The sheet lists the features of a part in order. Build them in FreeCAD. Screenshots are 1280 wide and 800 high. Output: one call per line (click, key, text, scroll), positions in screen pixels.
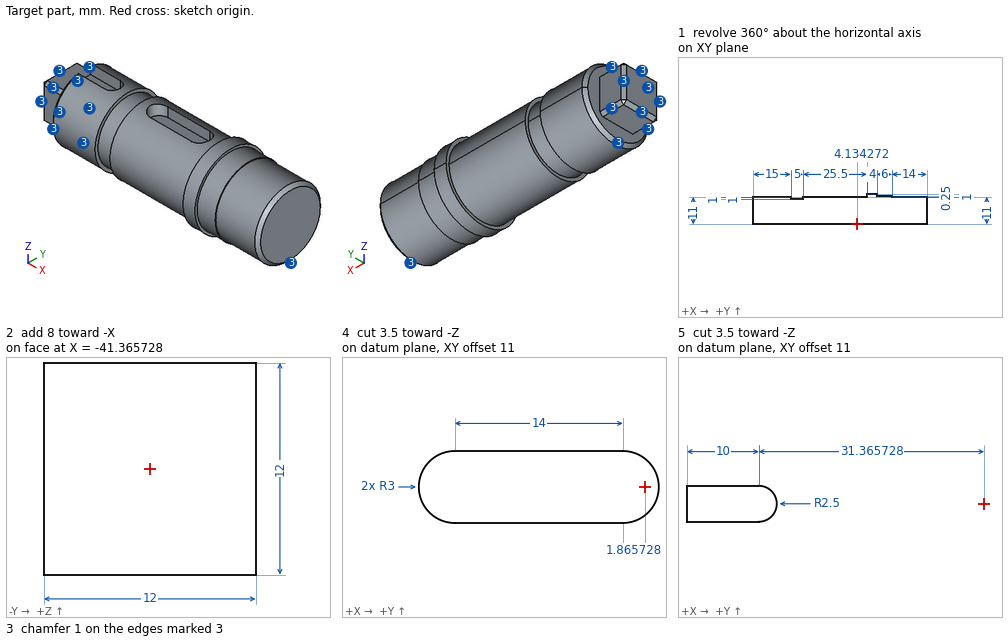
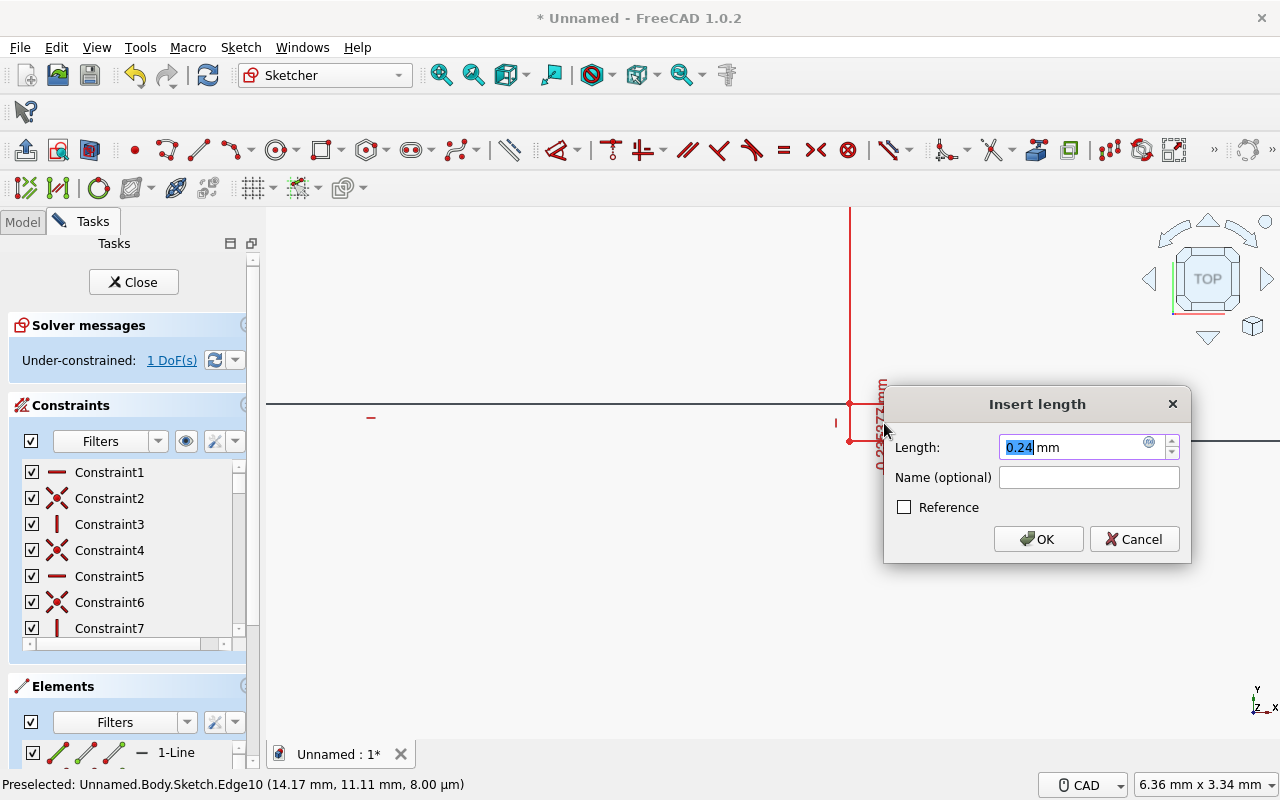
text(0.25)
key(Return)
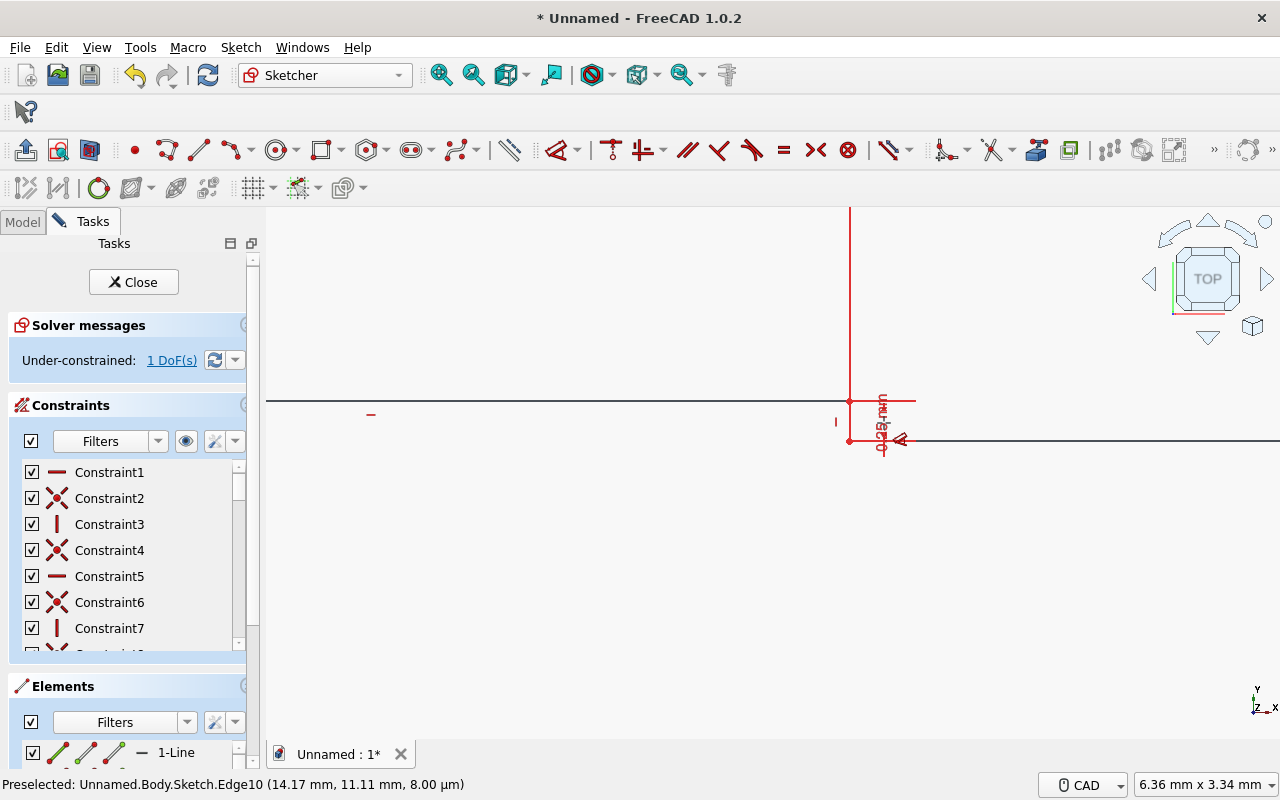
scroll(871, 433, down, 15)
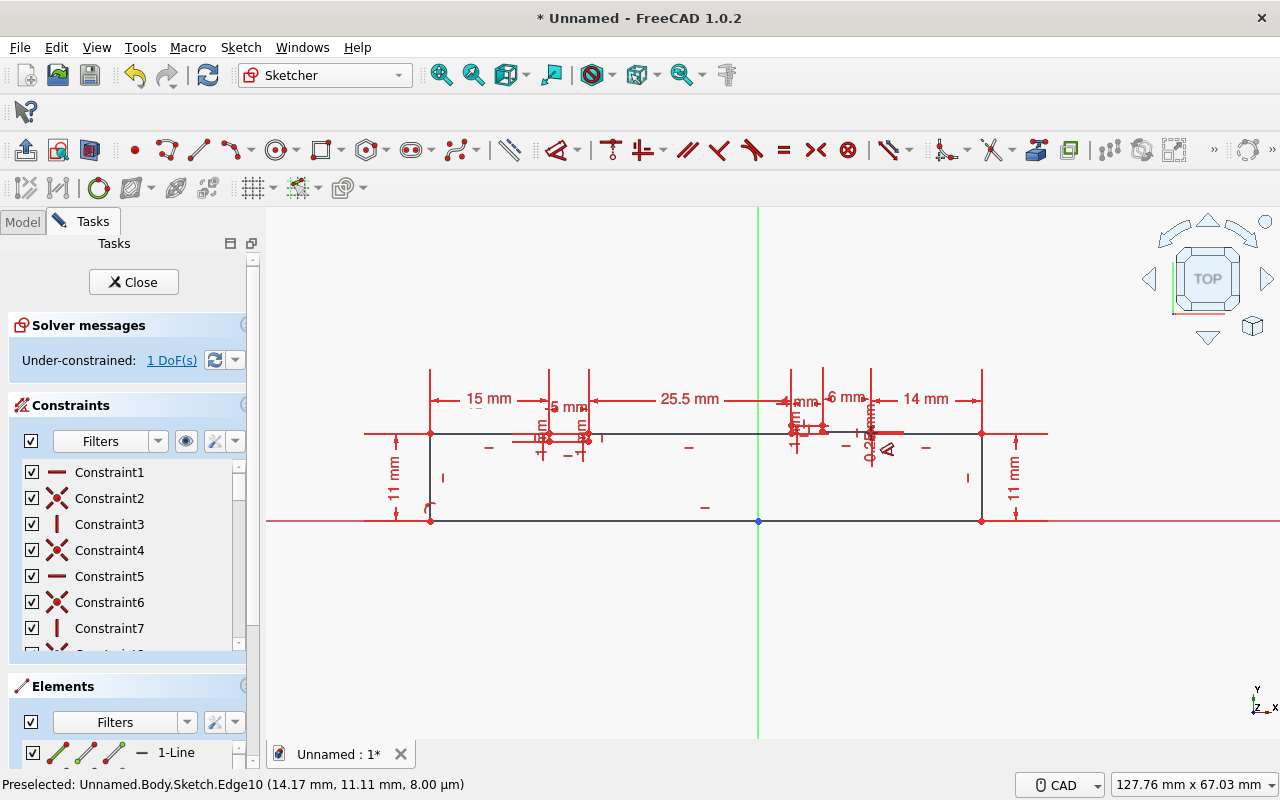
scroll(791, 434, up, 3)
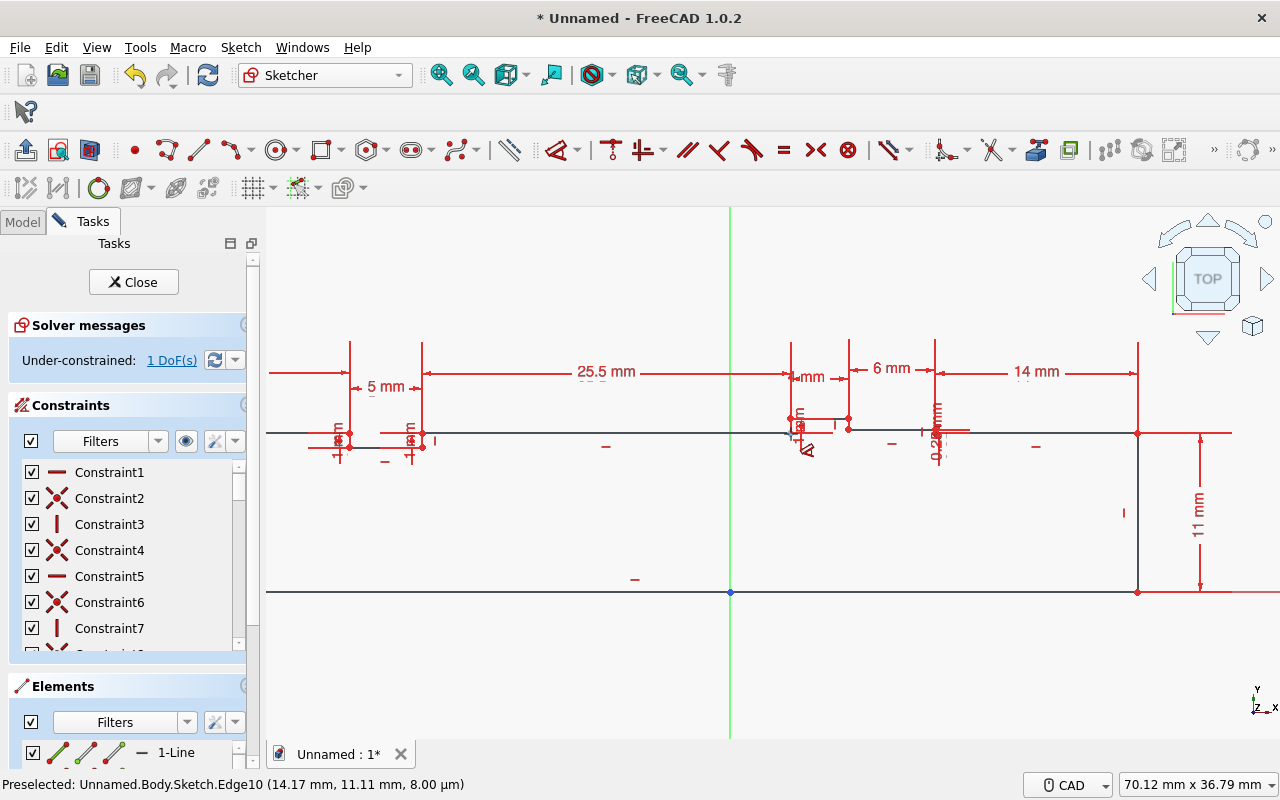
click(791, 433)
click(761, 626)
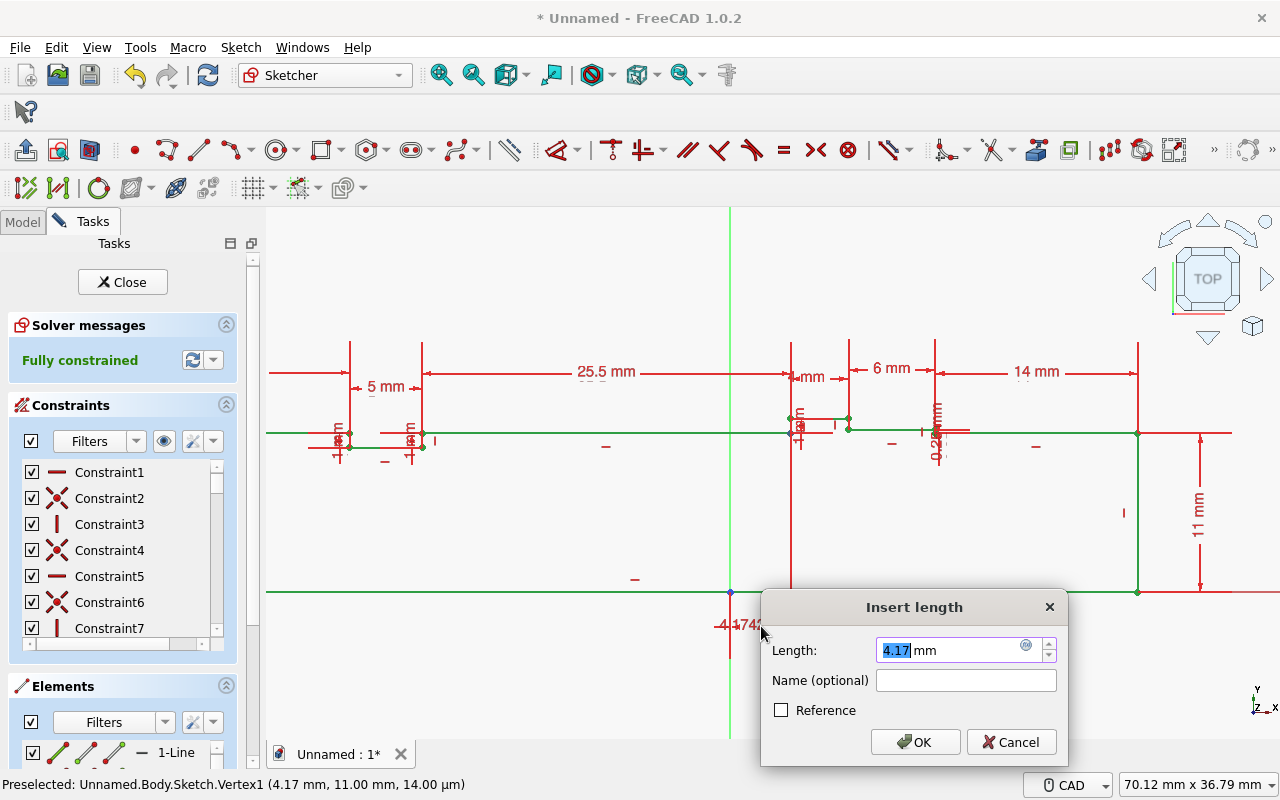
text(4.134272)
key(Return)
key(Escape)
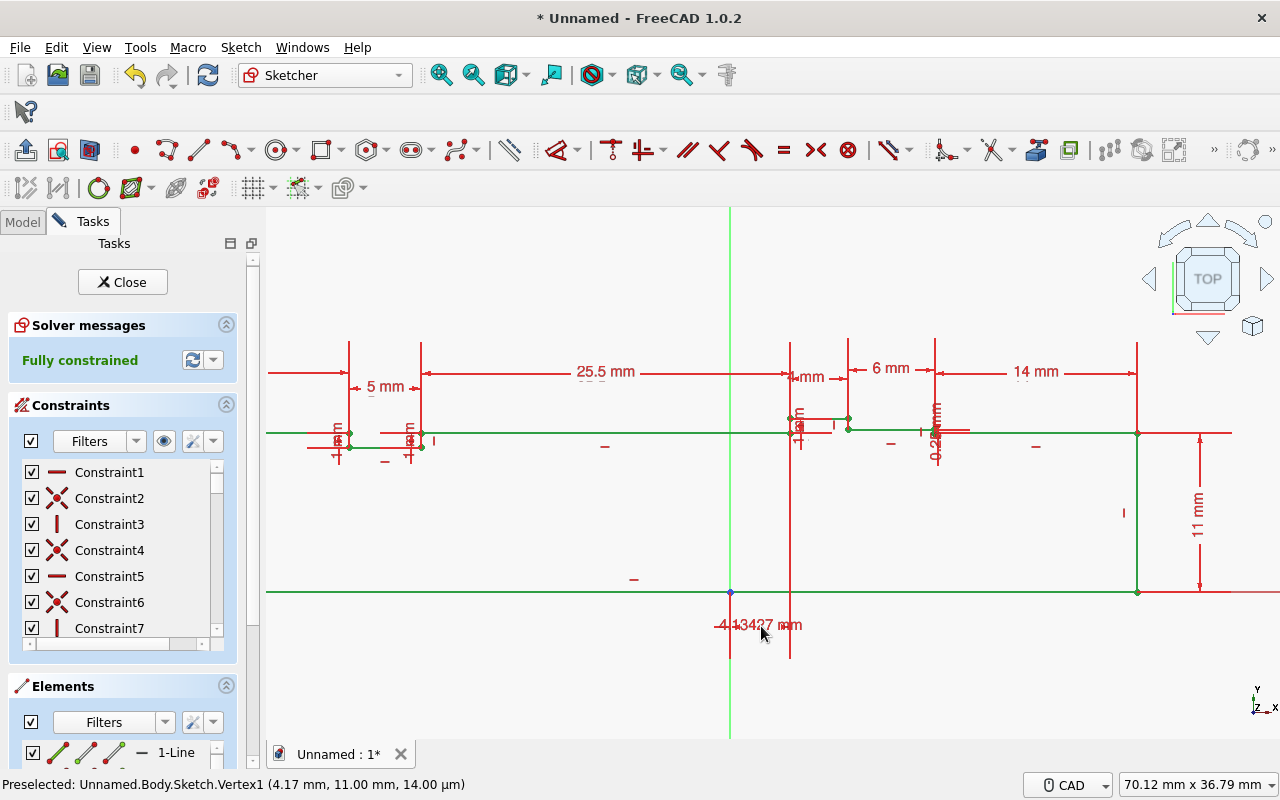
click(123, 282)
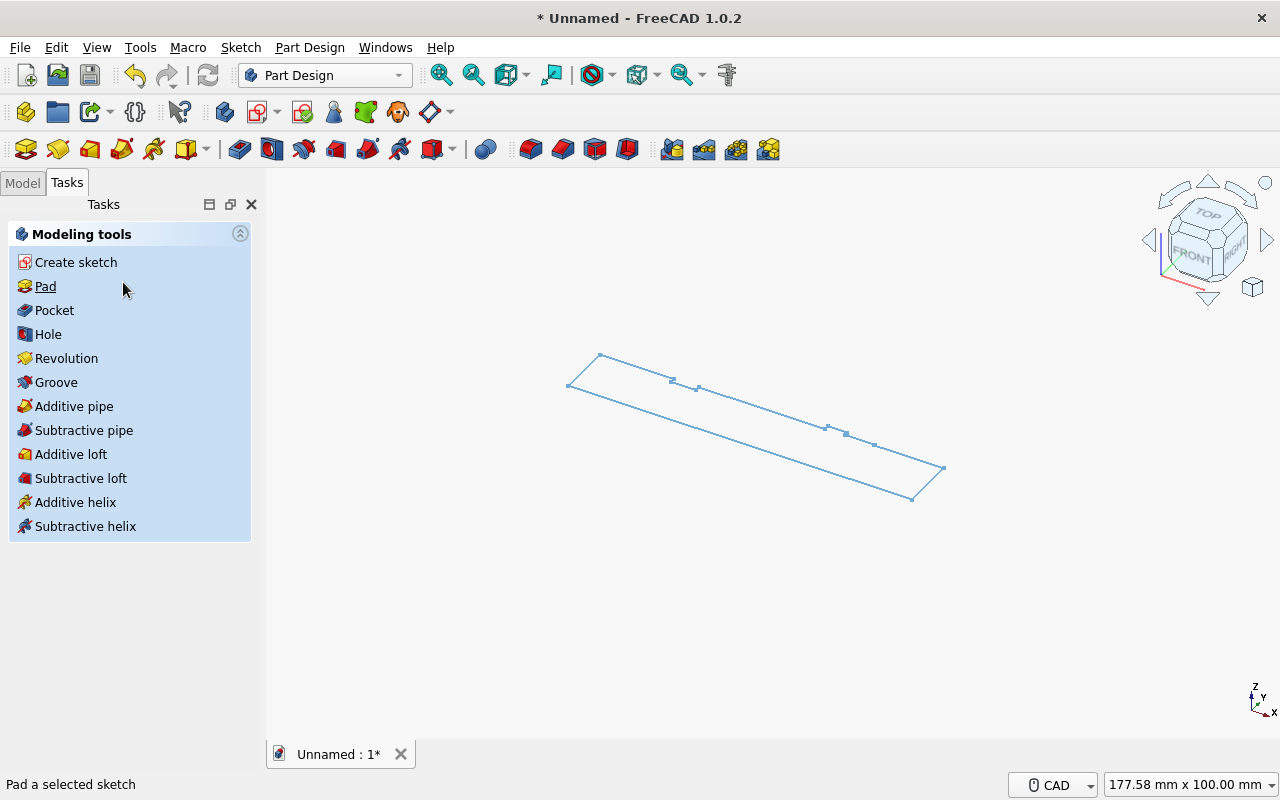
click(58, 150)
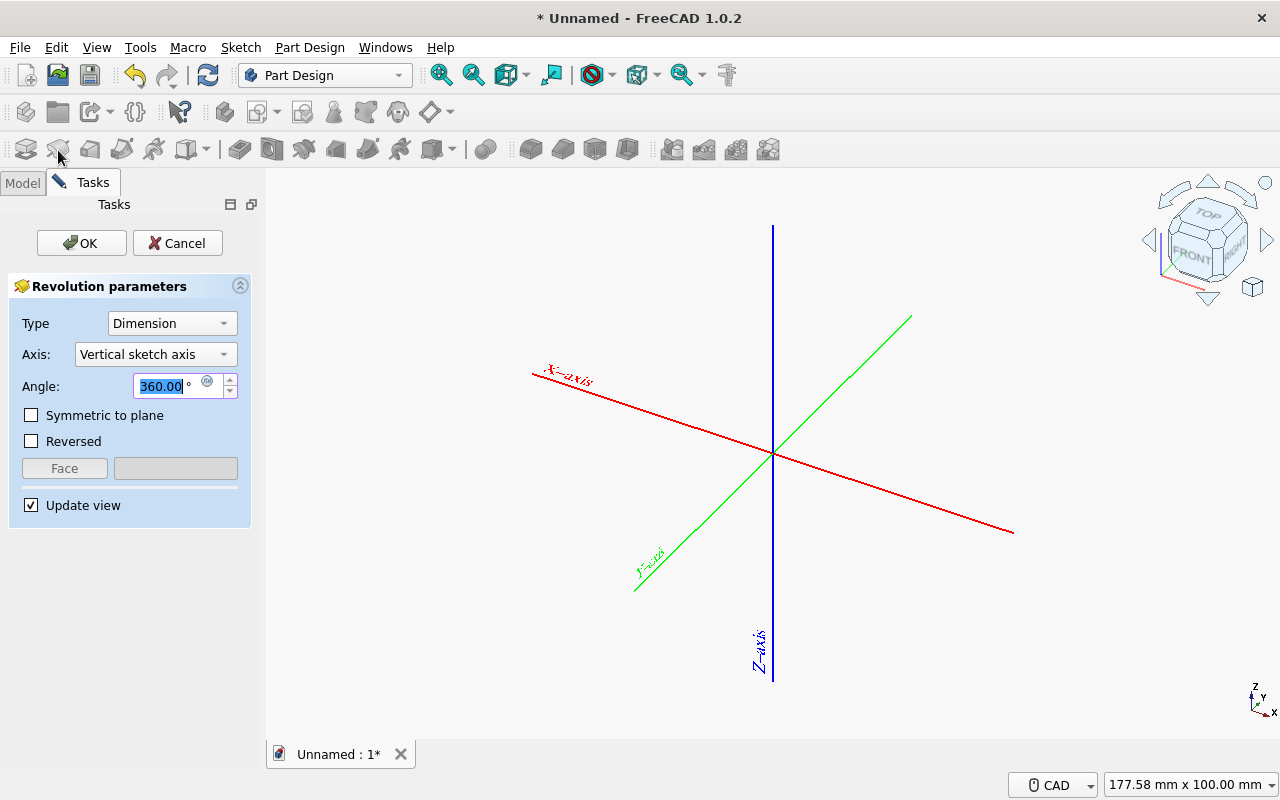
click(156, 354)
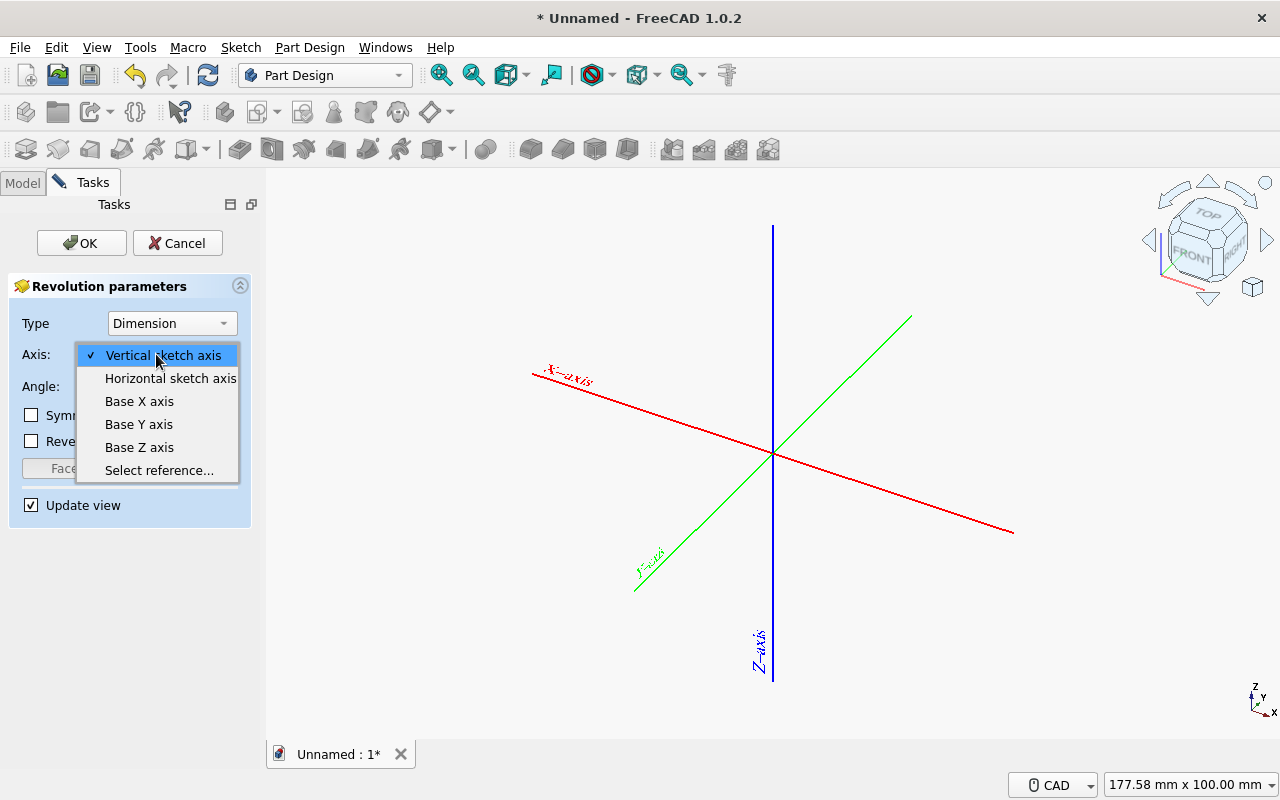
click(156, 378)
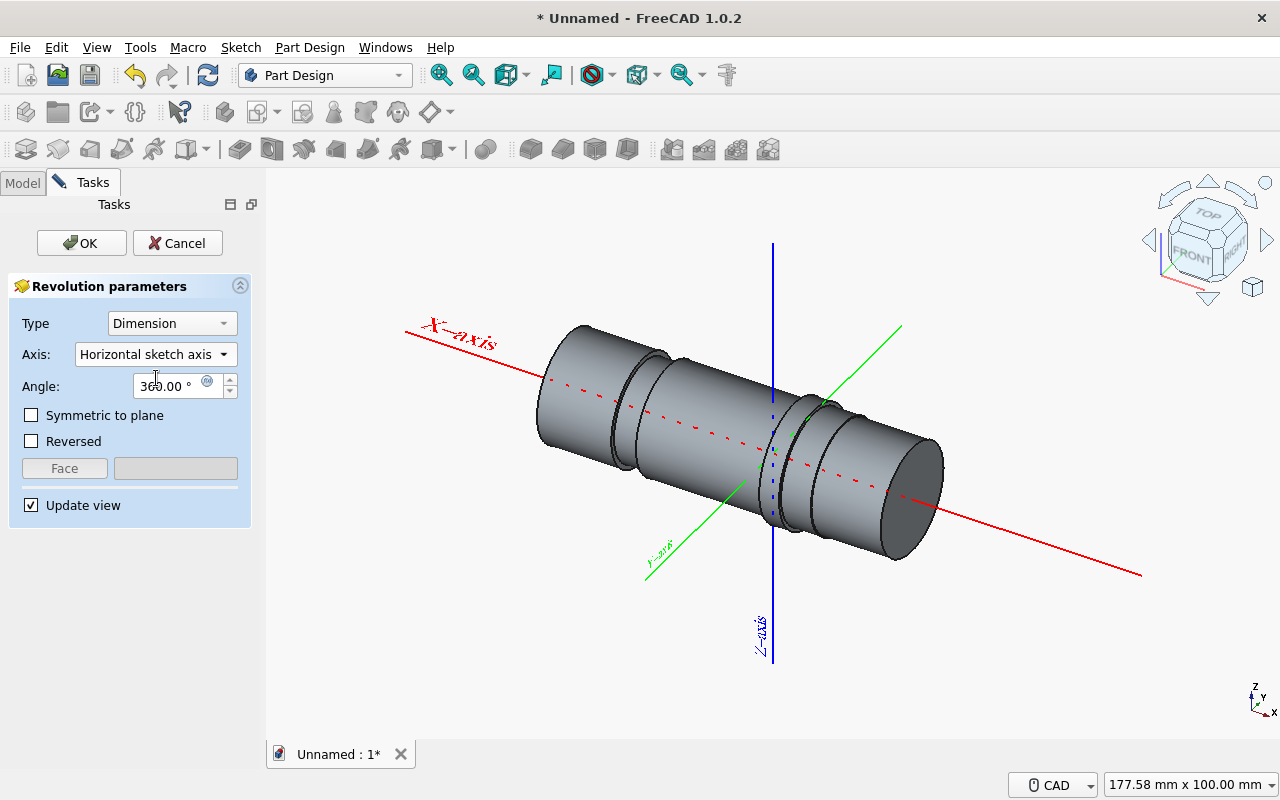
click(82, 243)